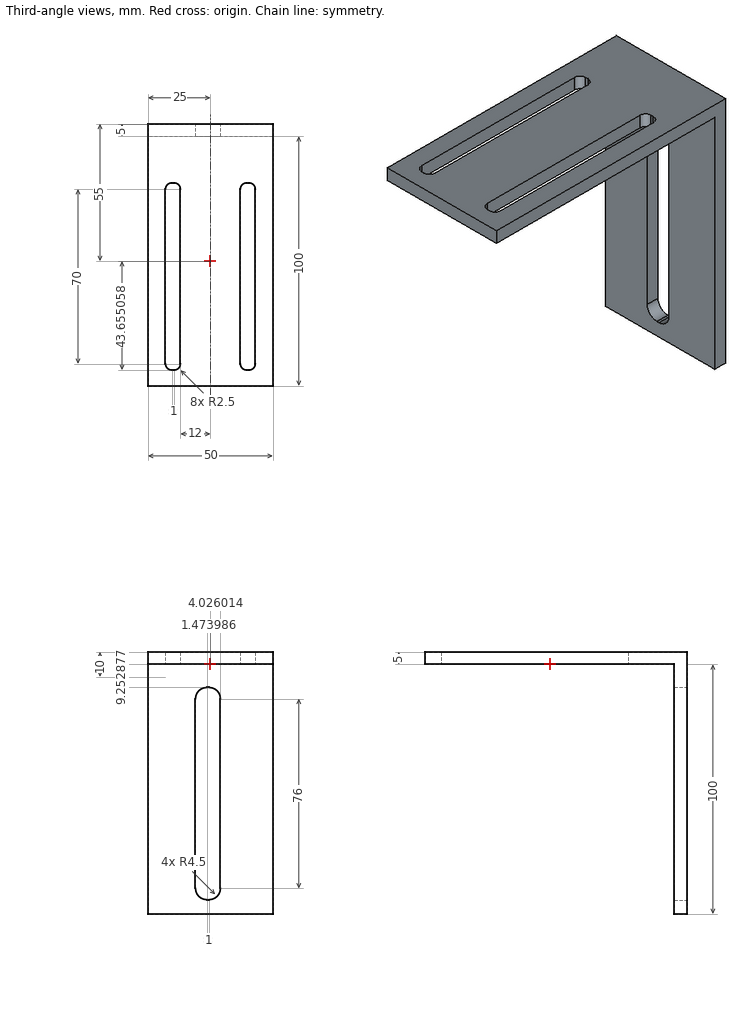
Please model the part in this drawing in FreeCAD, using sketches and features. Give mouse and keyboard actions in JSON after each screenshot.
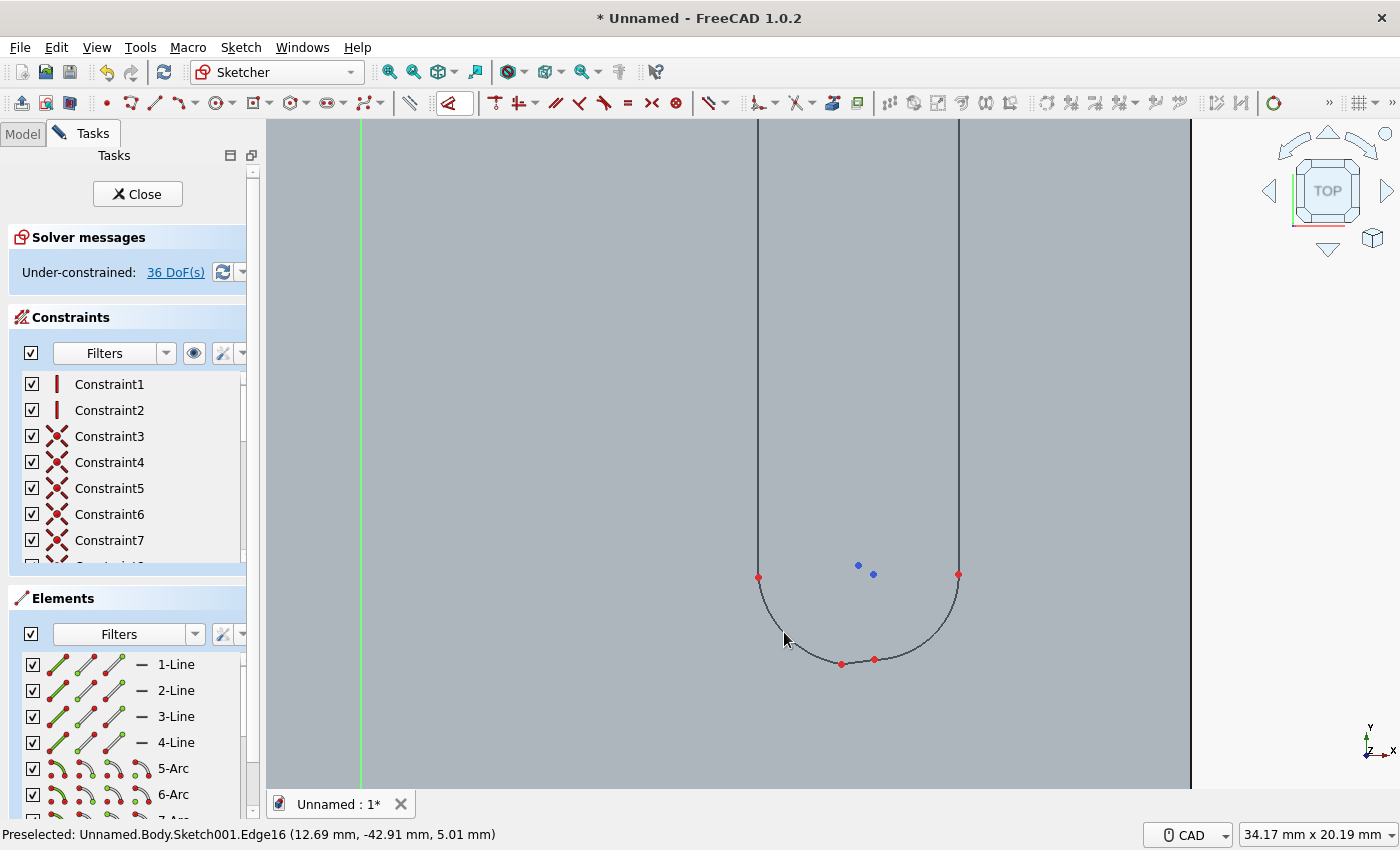
{"action": "scroll", "coordinate": [844, 660], "scroll_direction": "down", "scroll_amount": 9}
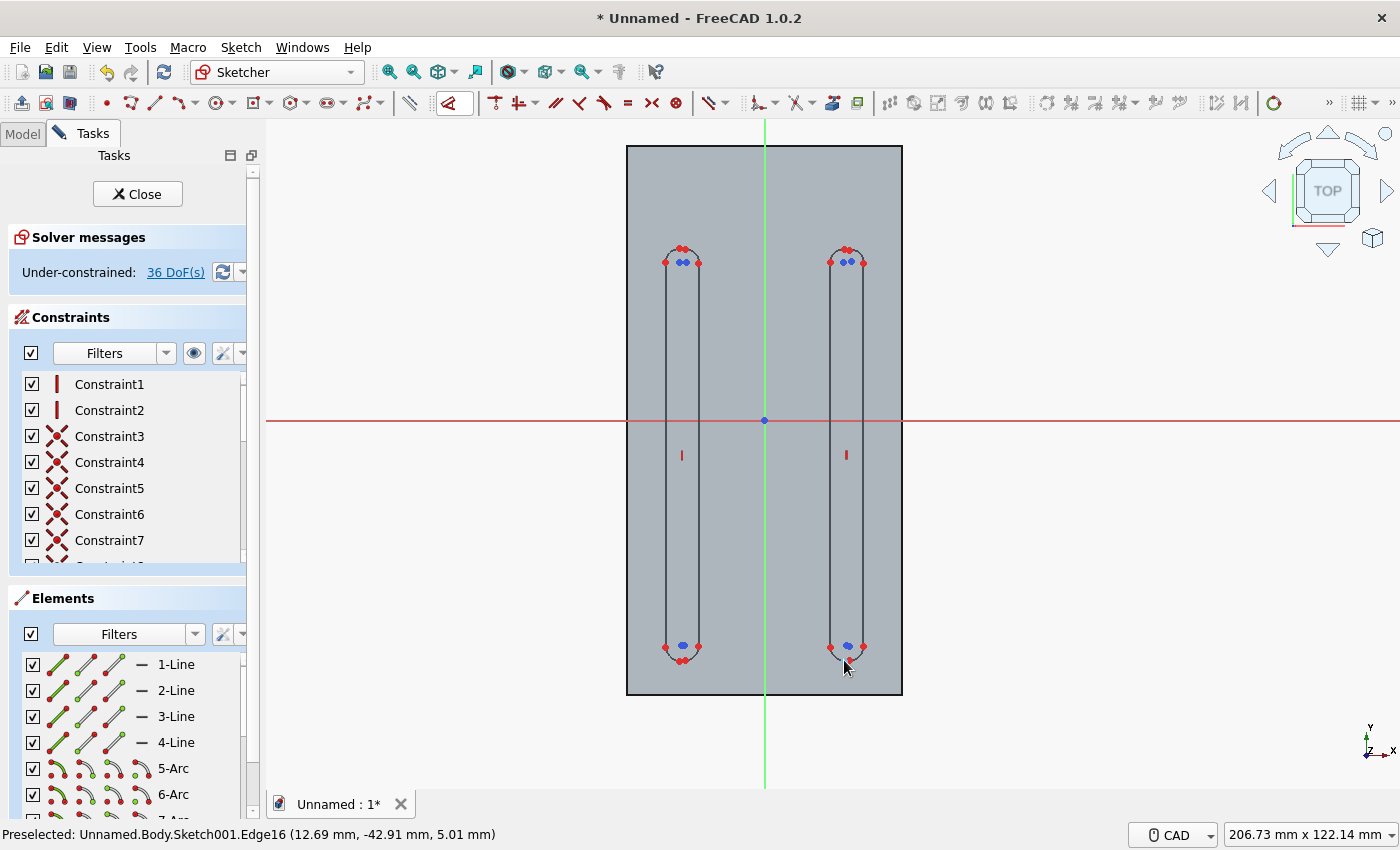
{"action": "scroll", "coordinate": [681, 661], "scroll_direction": "up", "scroll_amount": 11}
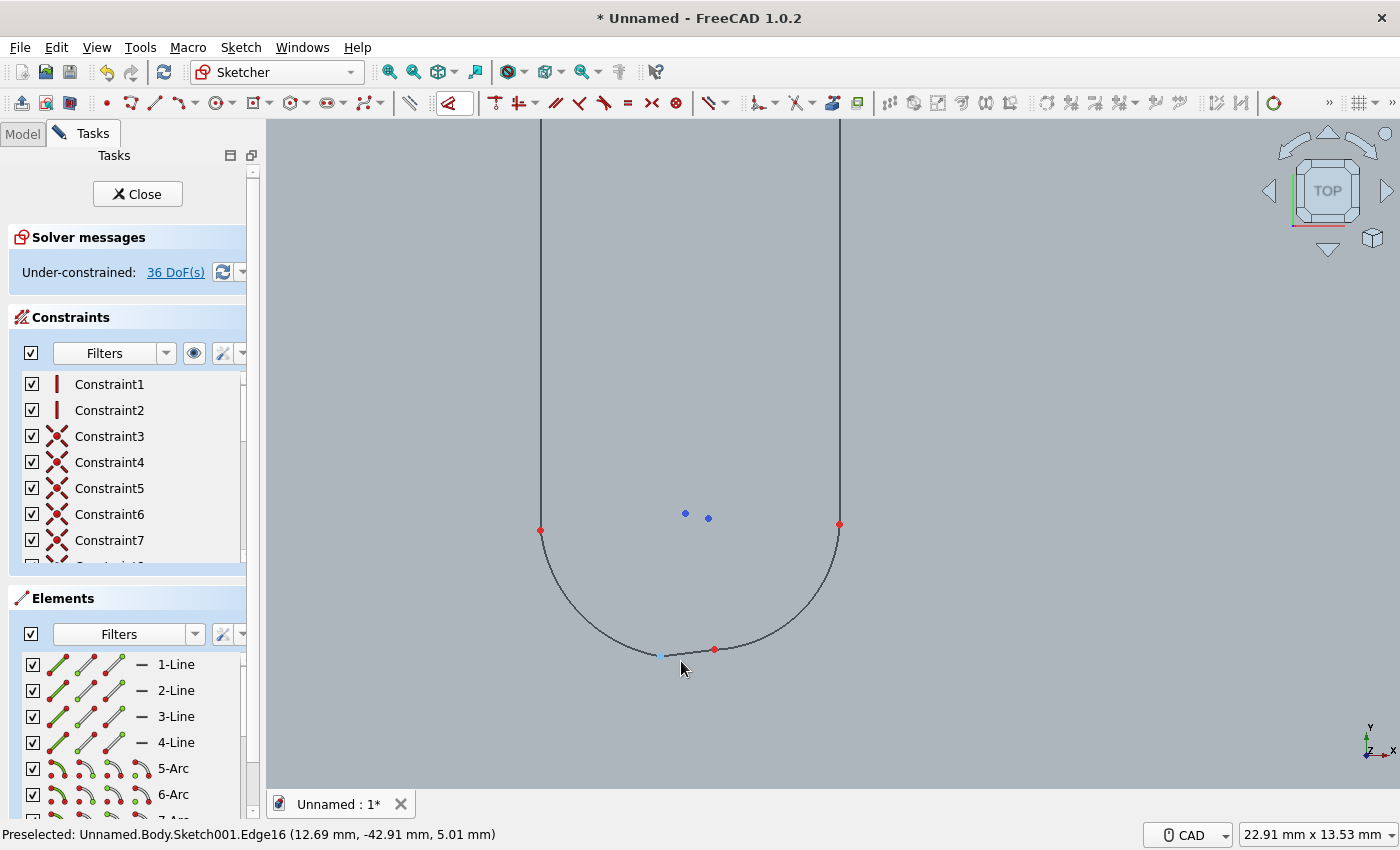
{"action": "left_click", "coordinate": [677, 654]}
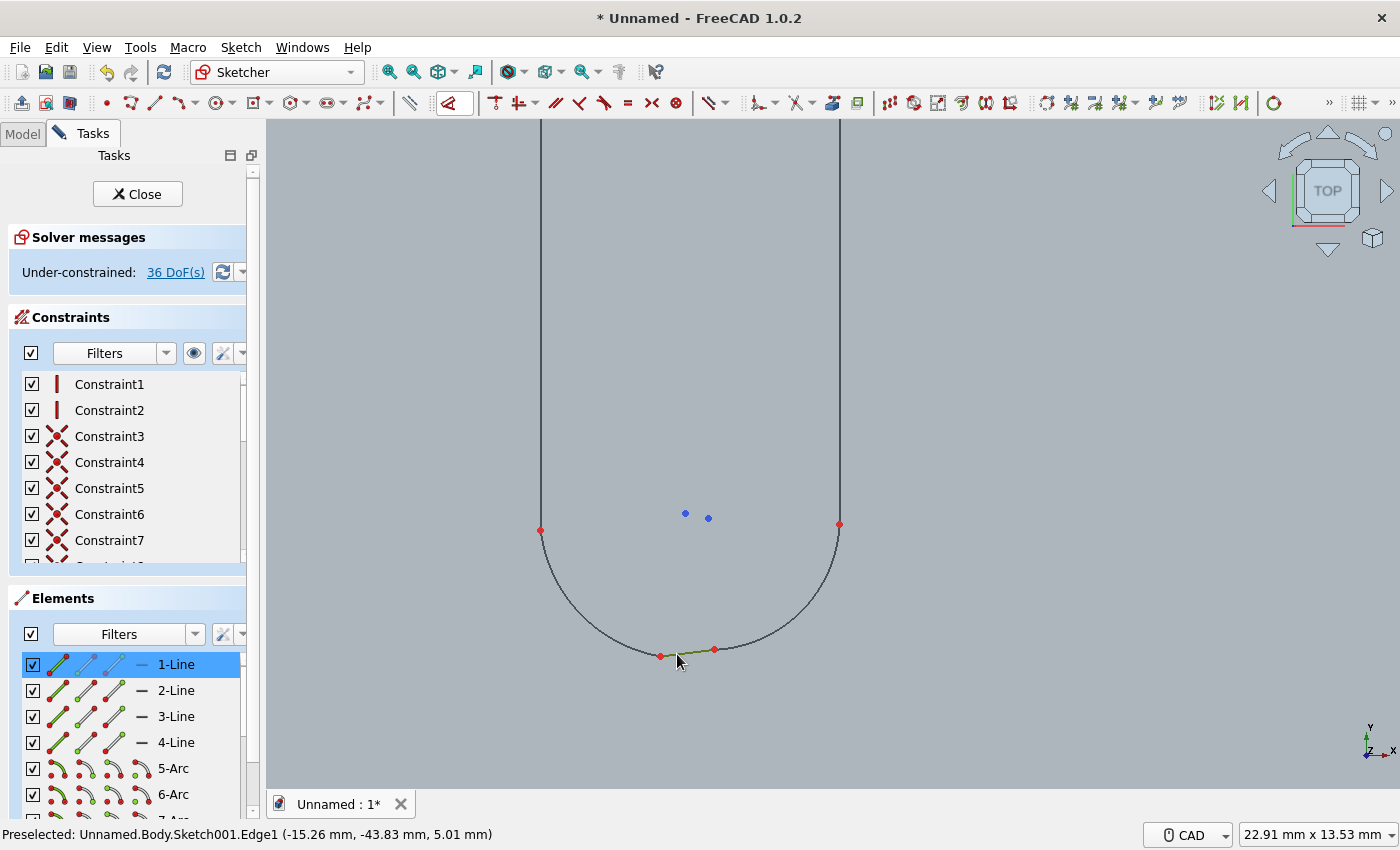
{"action": "scroll", "coordinate": [681, 661], "scroll_direction": "down", "scroll_amount": 11}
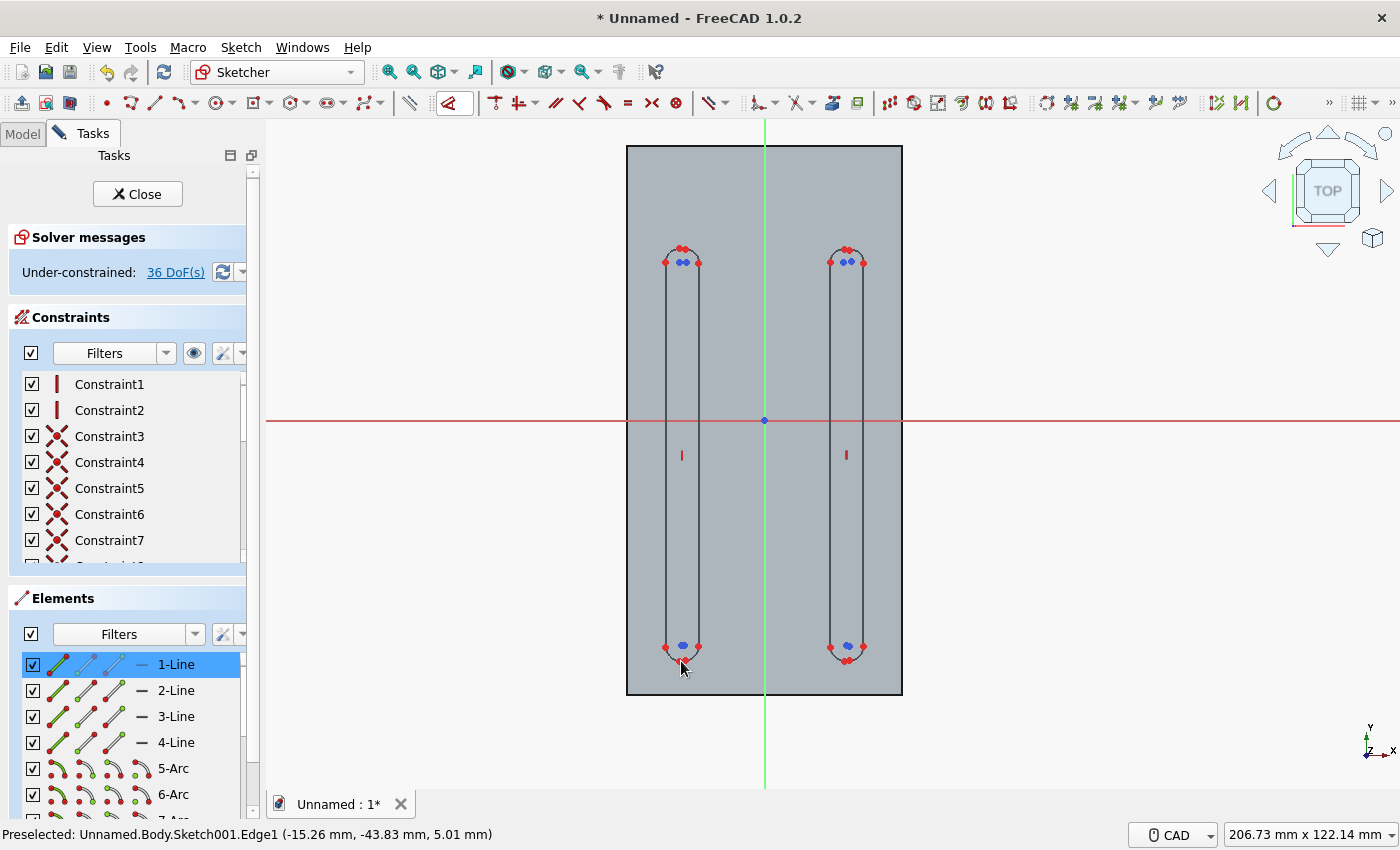
{"action": "scroll", "coordinate": [691, 659], "scroll_direction": "up", "scroll_amount": 4}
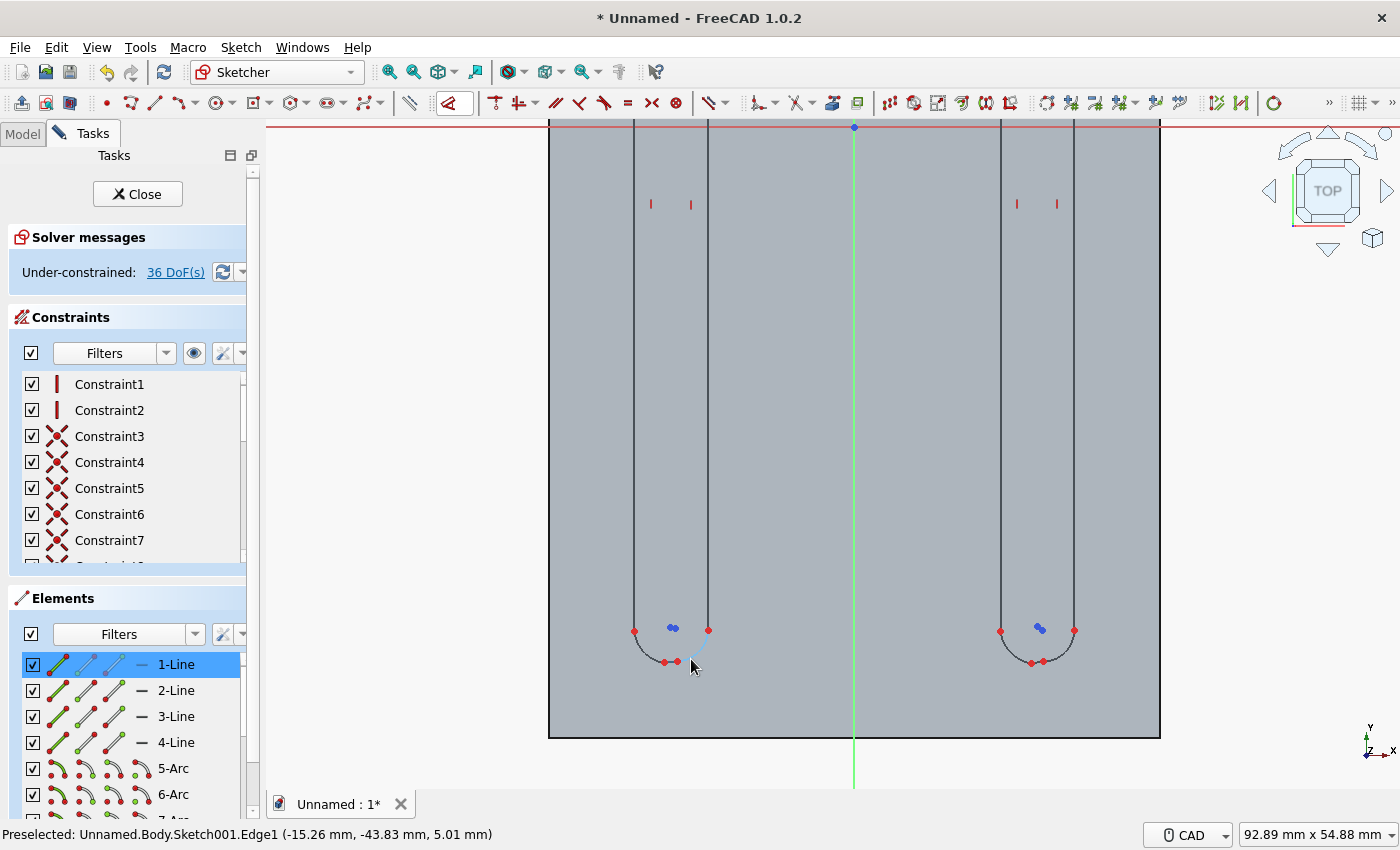
{"action": "left_click", "coordinate": [691, 658]}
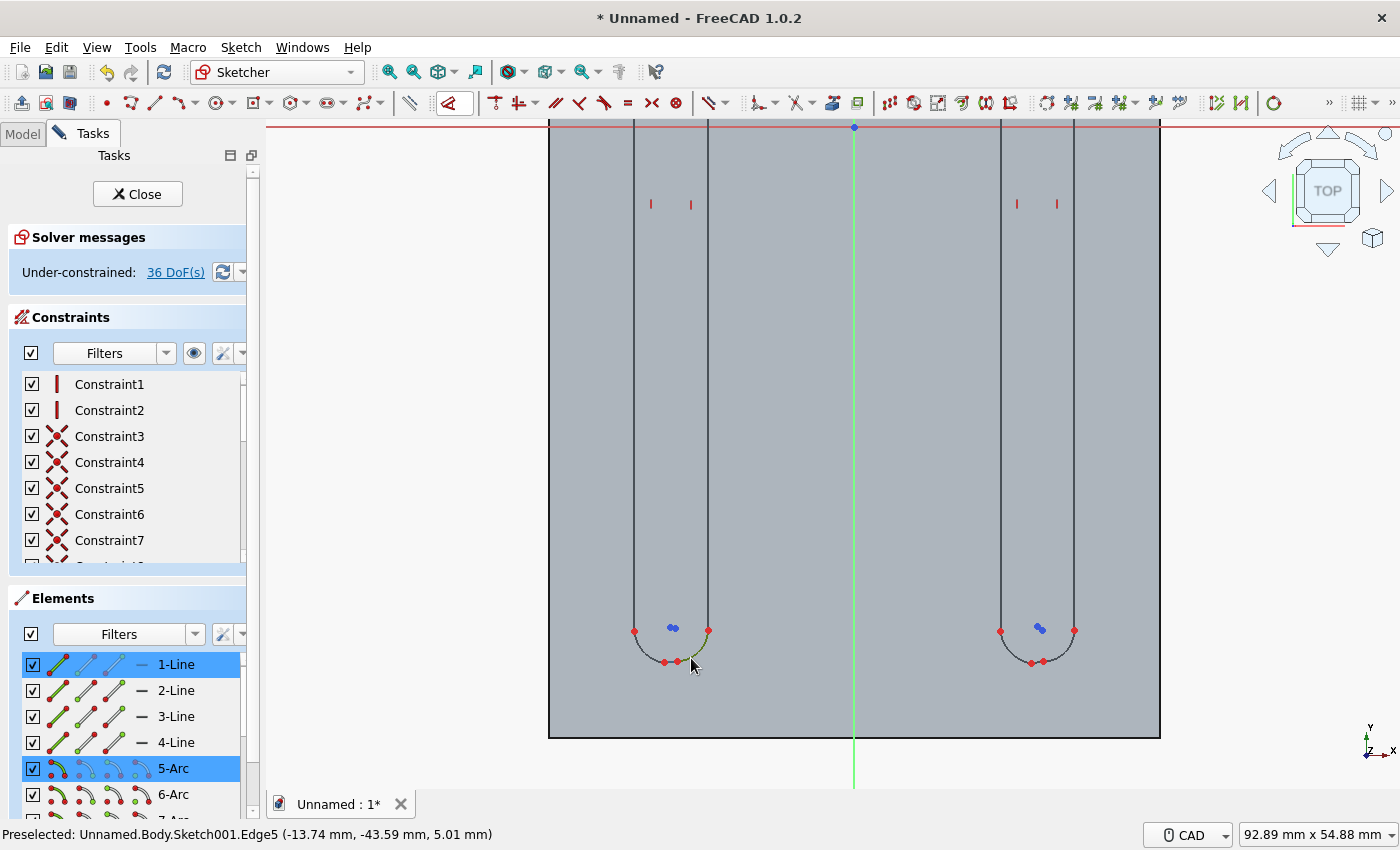
{"action": "left_click", "coordinate": [604, 104]}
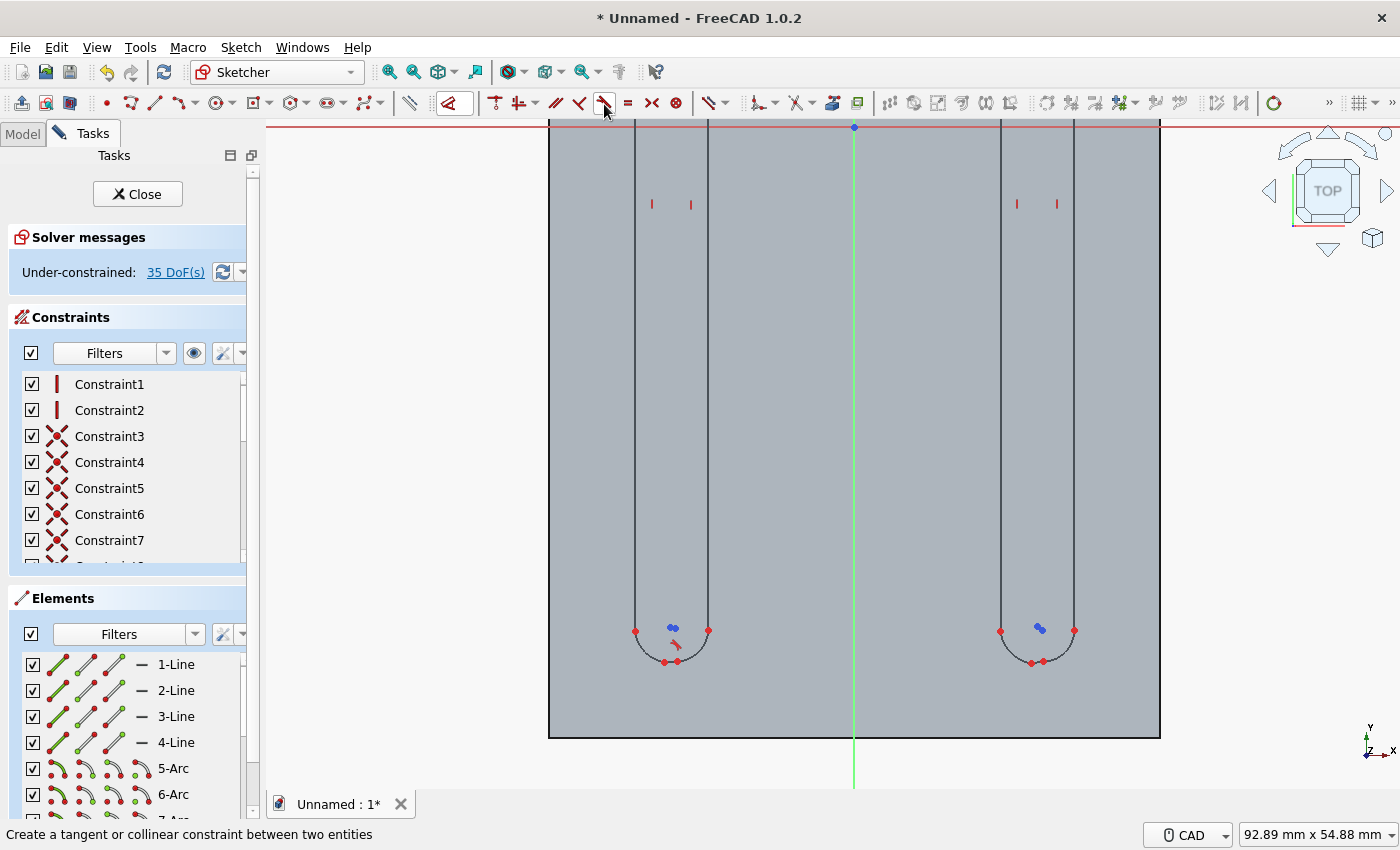
{"action": "scroll", "coordinate": [671, 662], "scroll_direction": "up", "scroll_amount": 4}